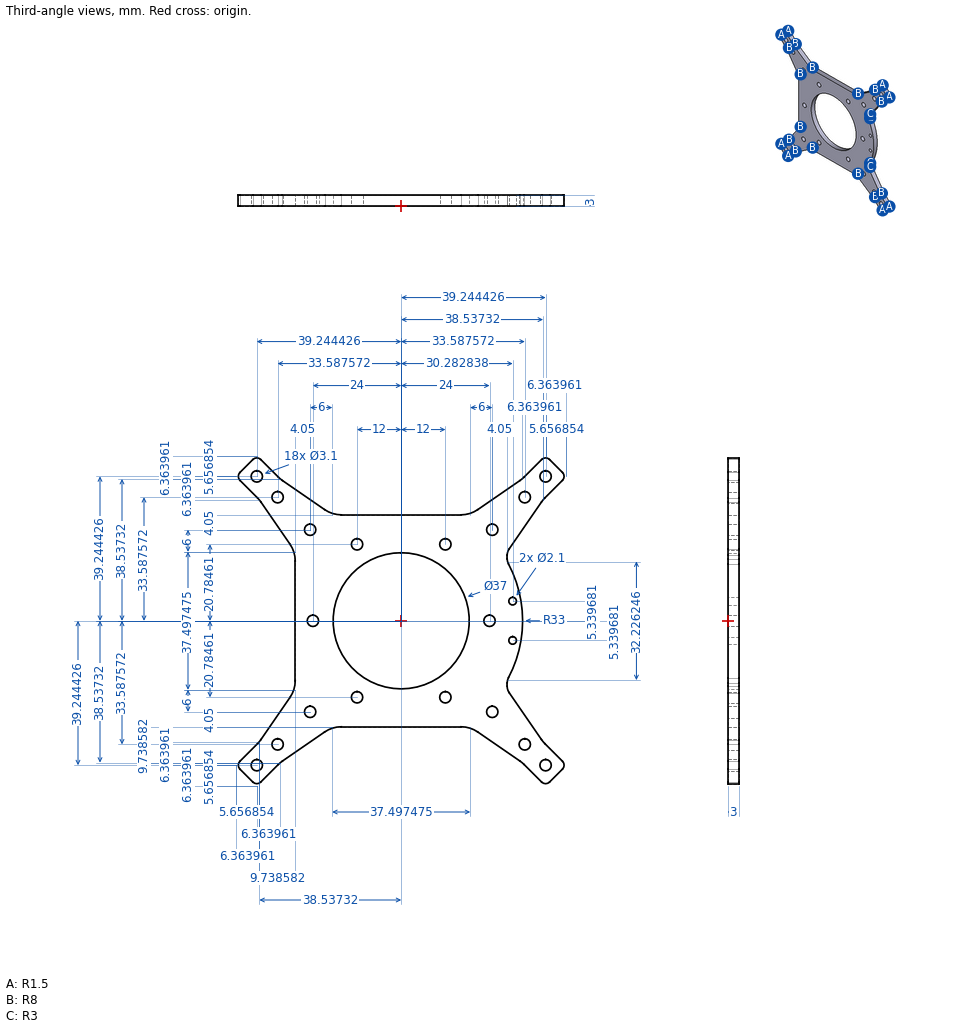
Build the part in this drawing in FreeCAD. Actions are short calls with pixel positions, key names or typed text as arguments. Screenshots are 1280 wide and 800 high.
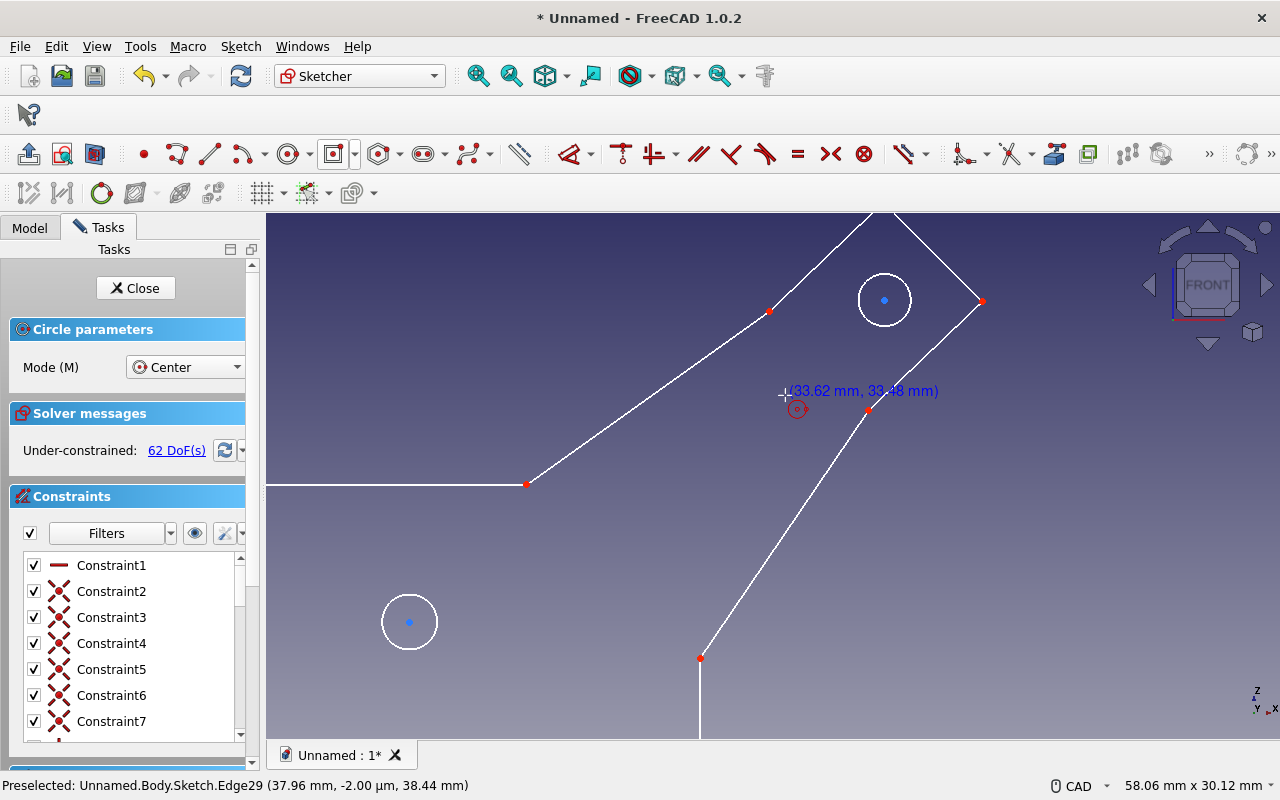
scroll(833, 348, down, 8)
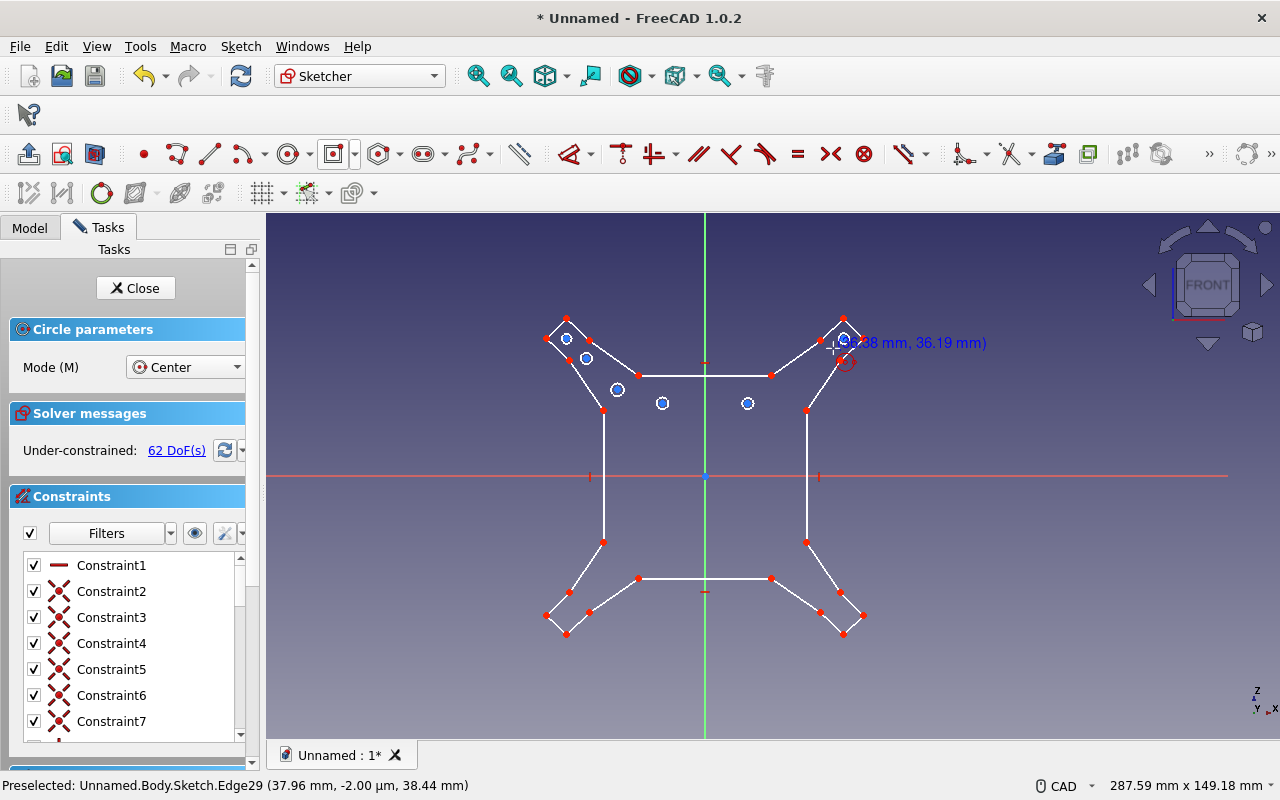
click(824, 358)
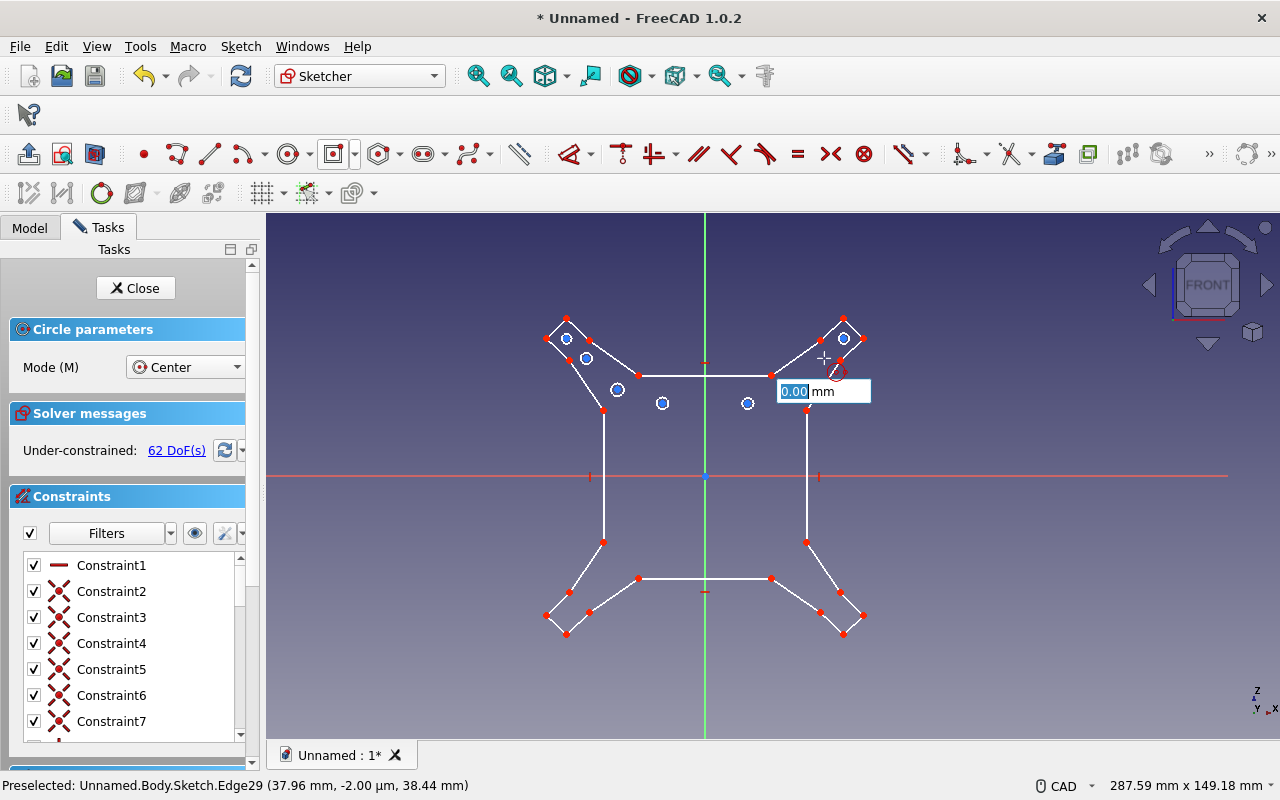
scroll(827, 354, up, 6)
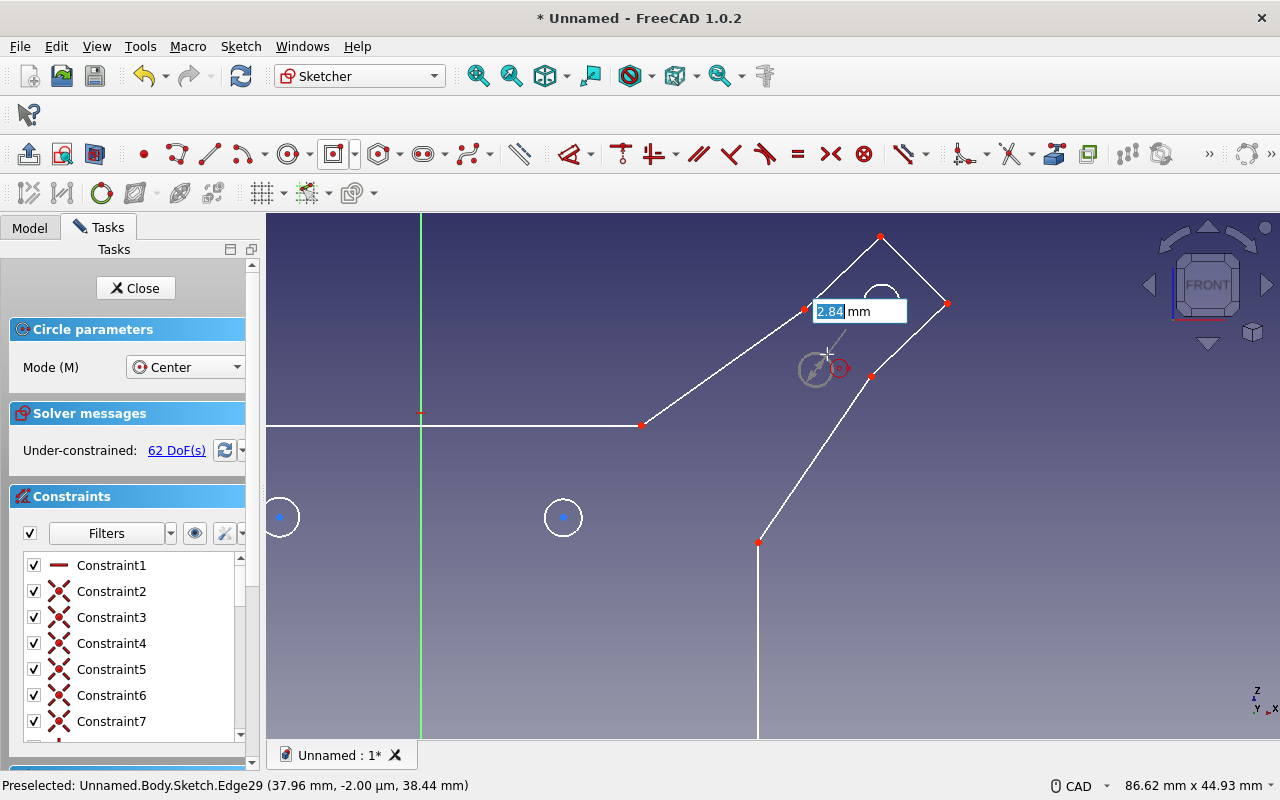
click(827, 352)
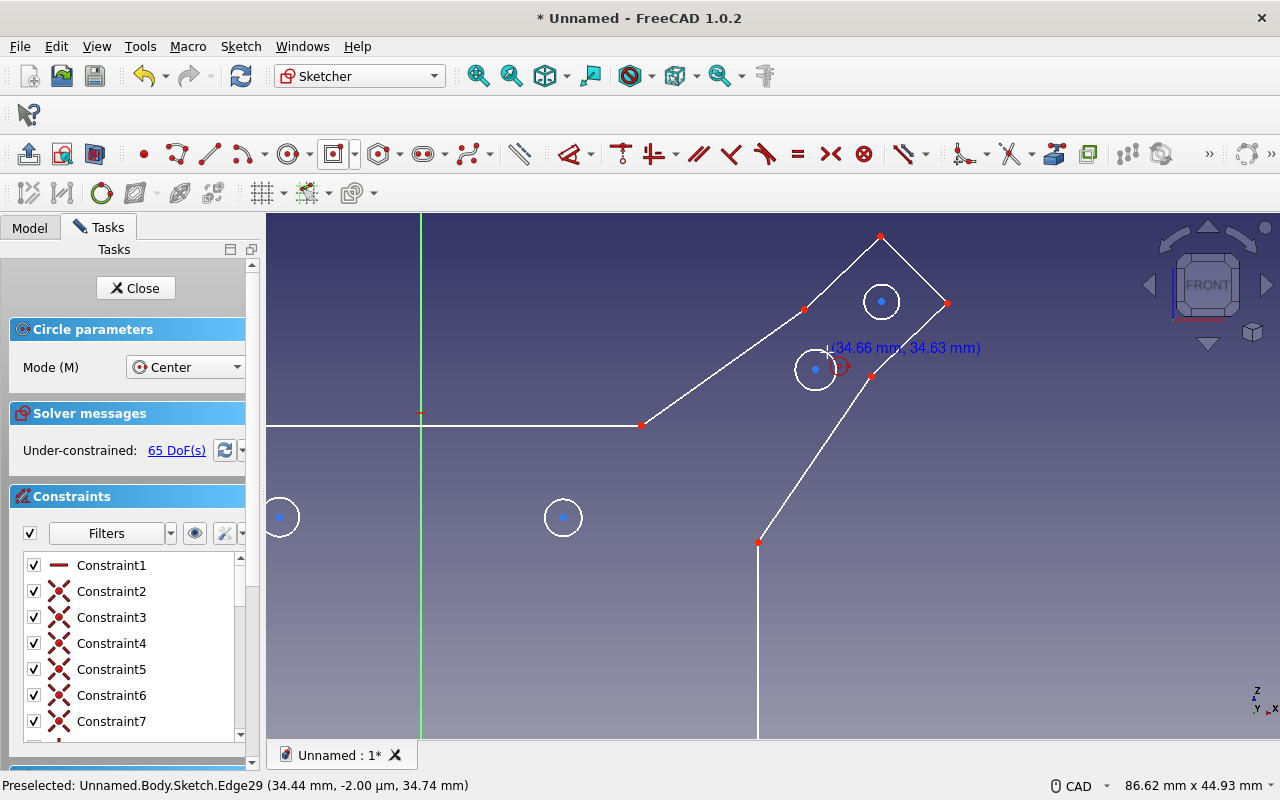
scroll(711, 469, up, 2)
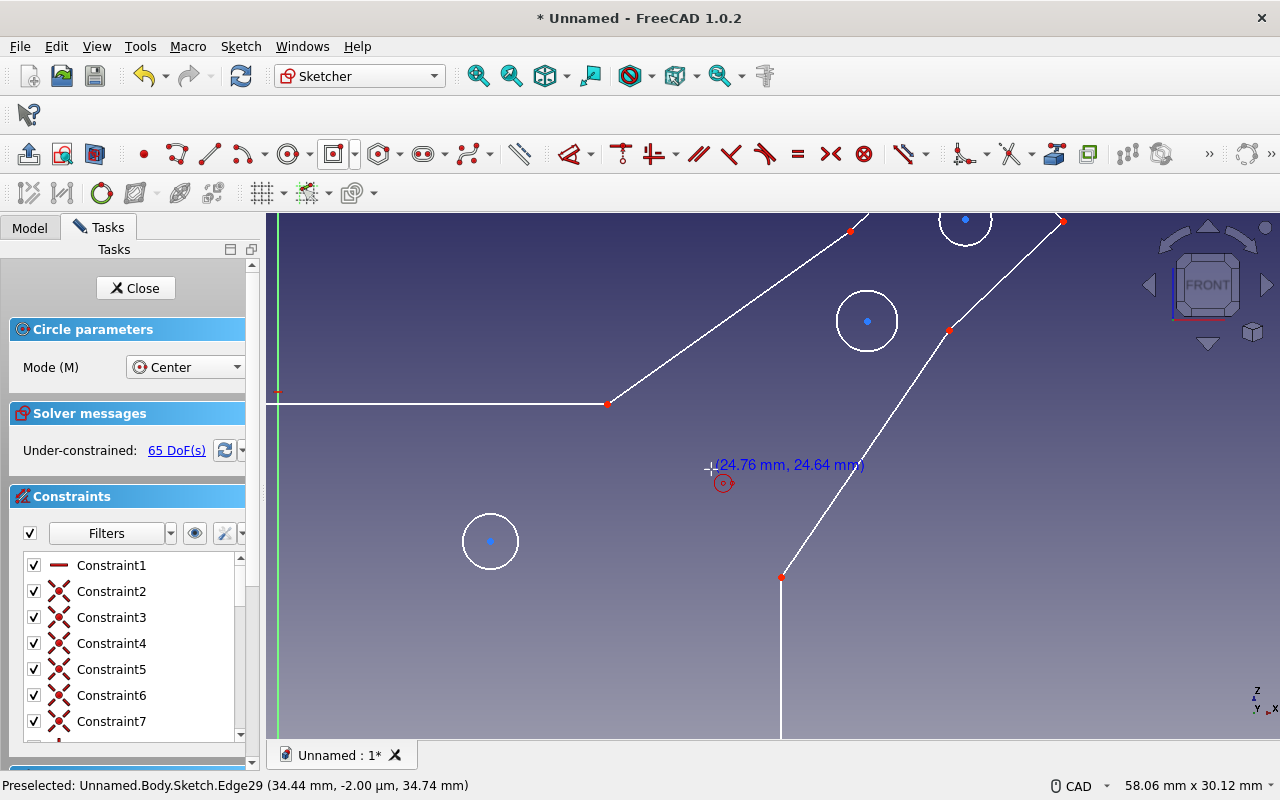
scroll(812, 369, down, 8)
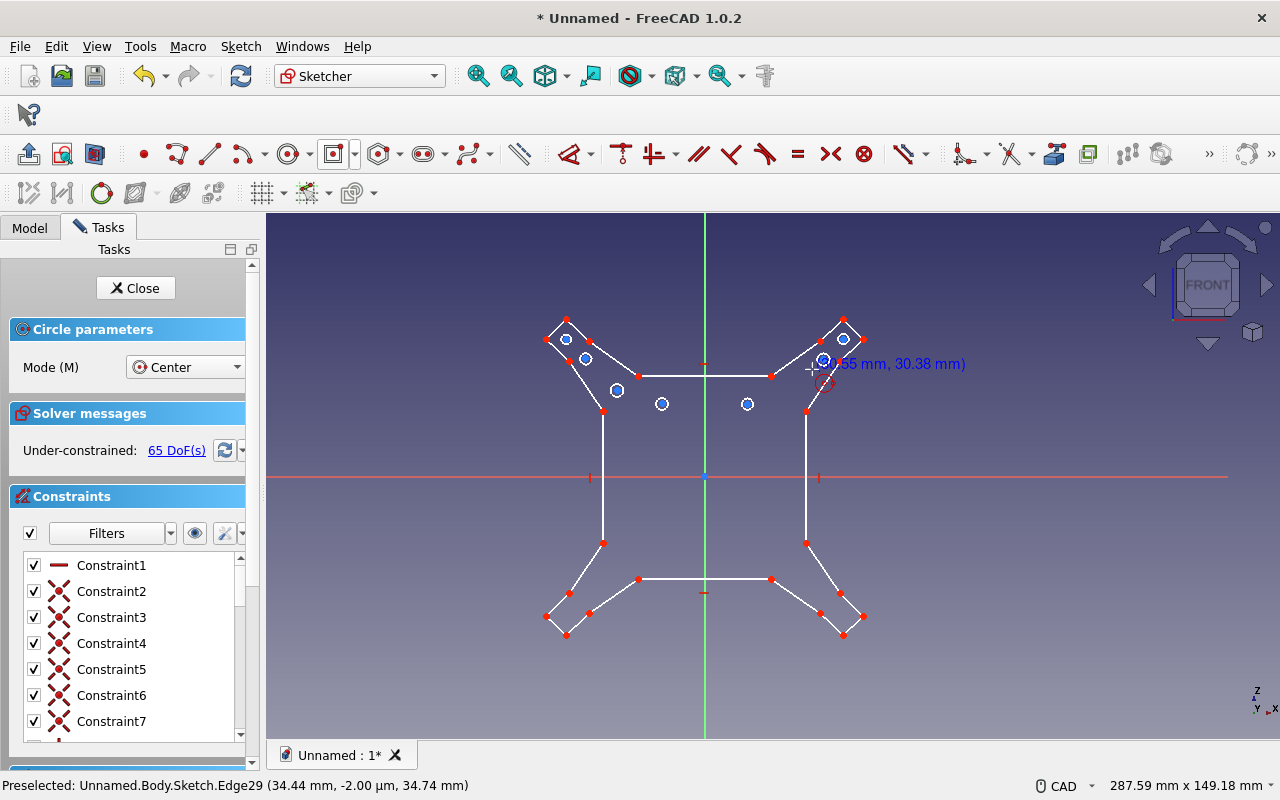
click(792, 389)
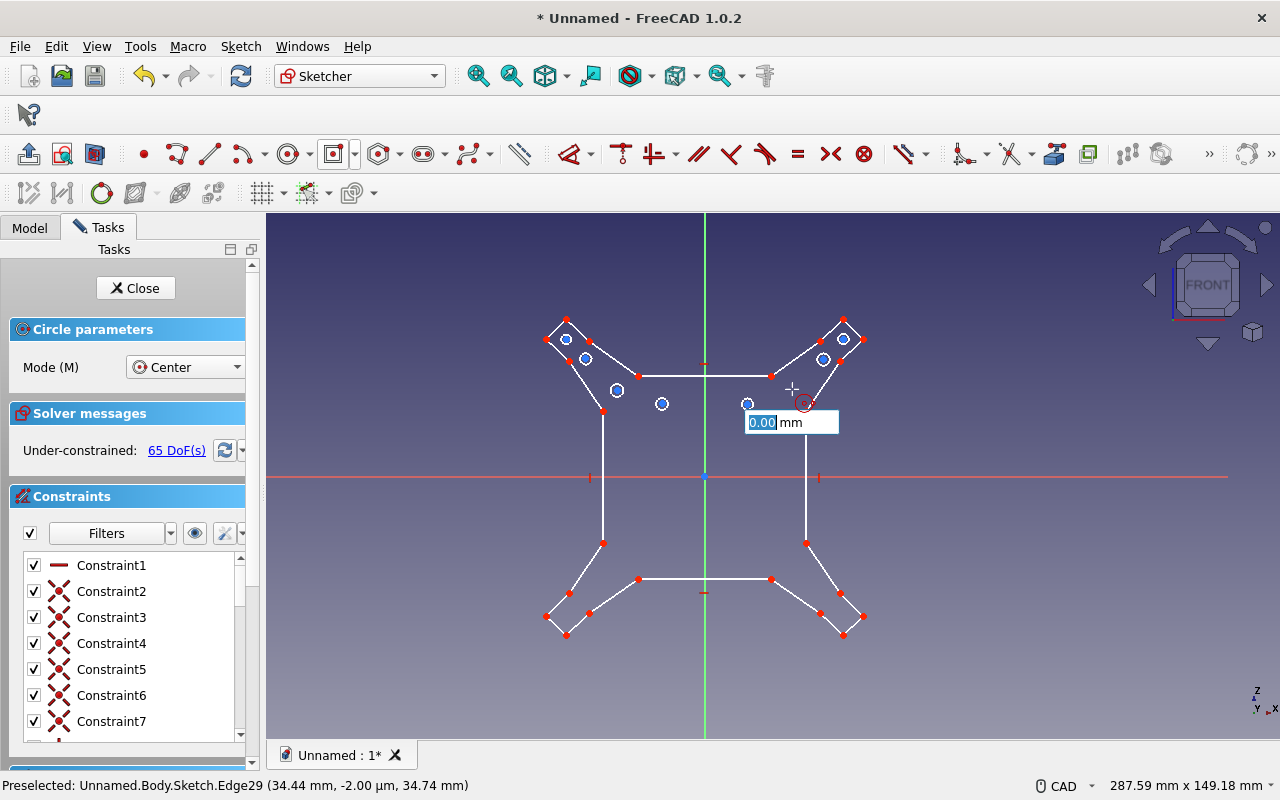
scroll(796, 385, up, 6)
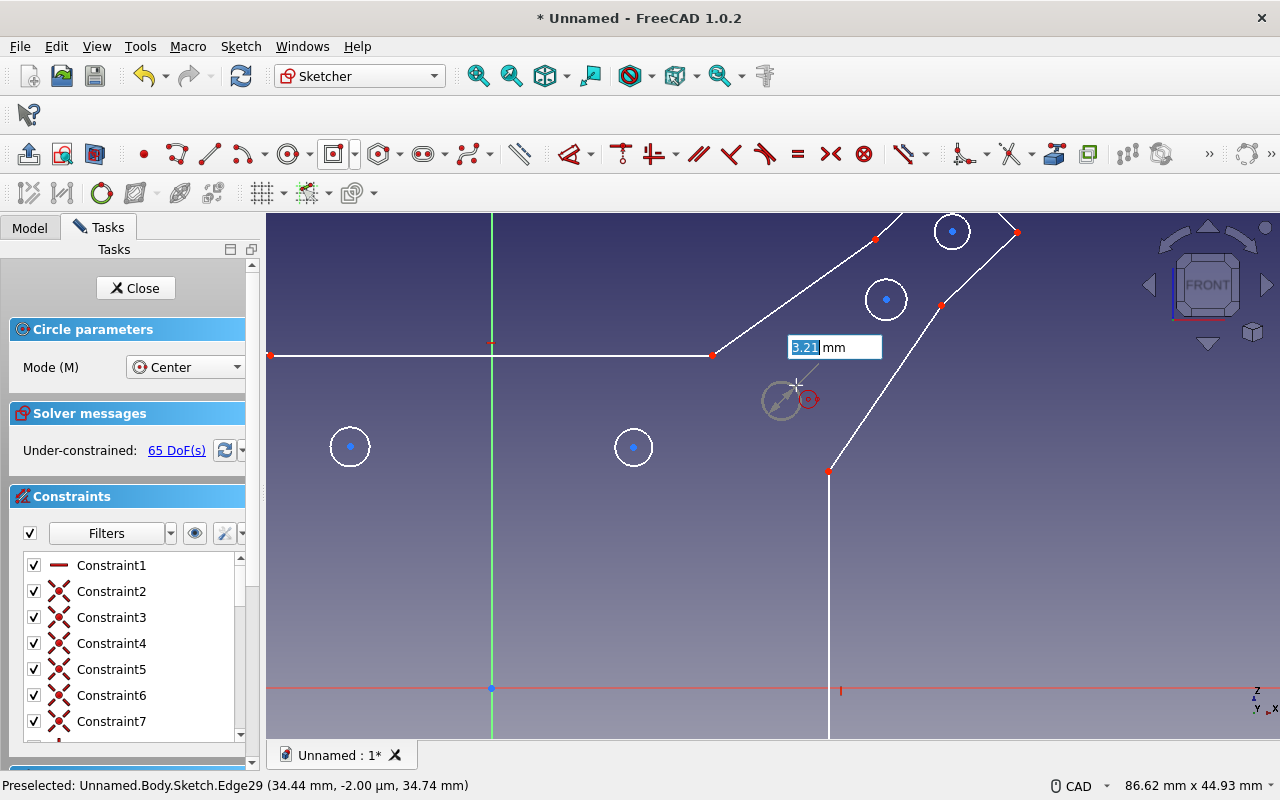
click(794, 386)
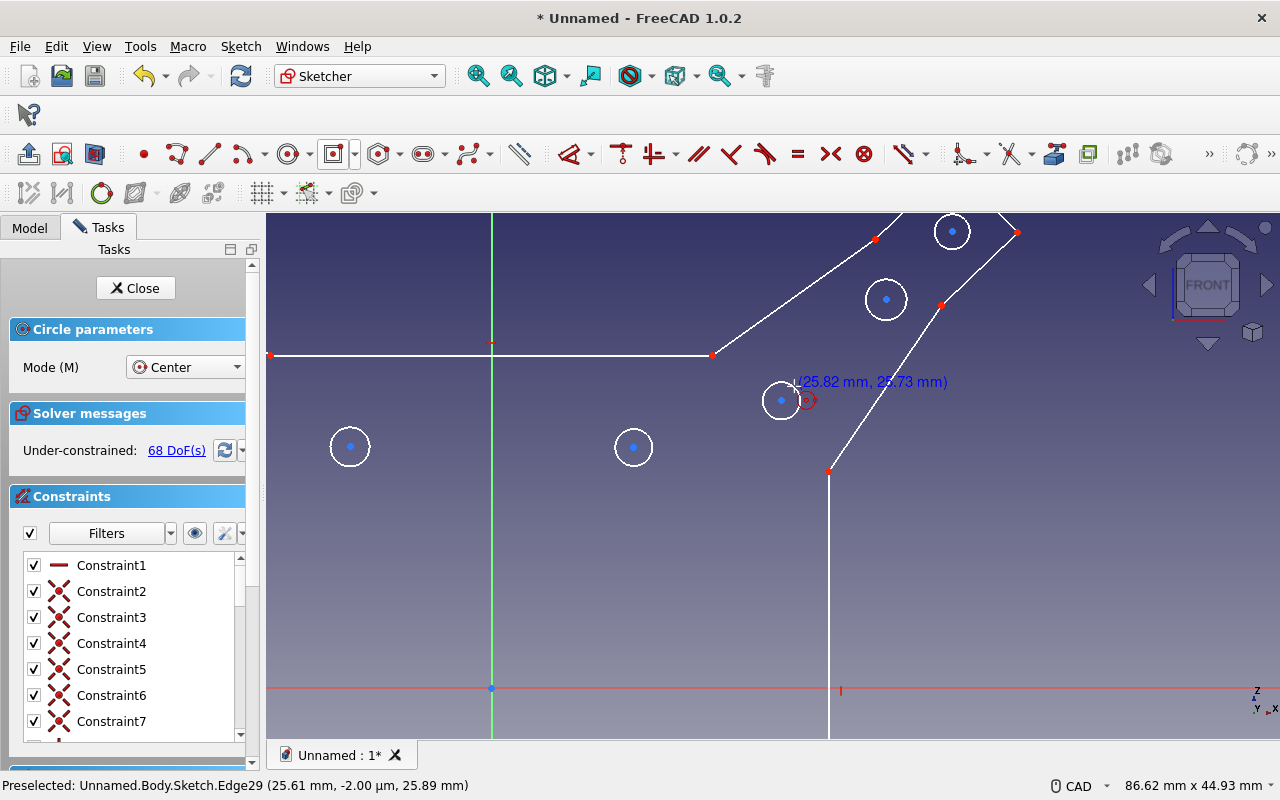
scroll(796, 385, down, 6)